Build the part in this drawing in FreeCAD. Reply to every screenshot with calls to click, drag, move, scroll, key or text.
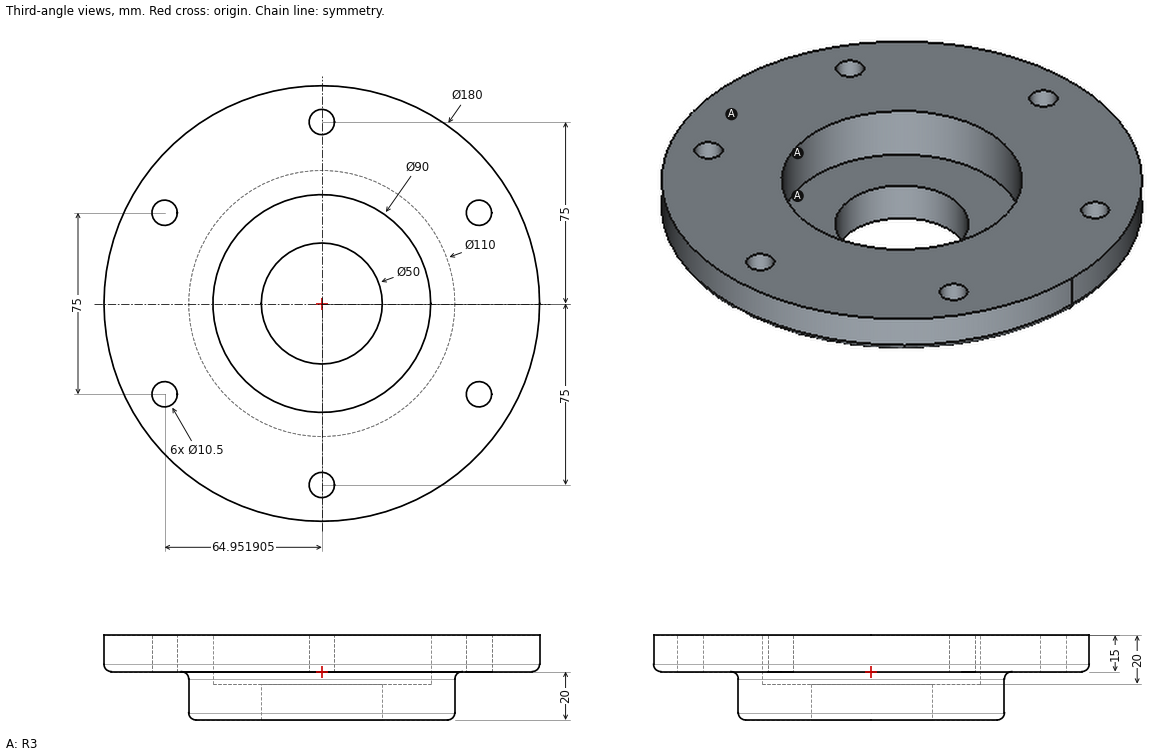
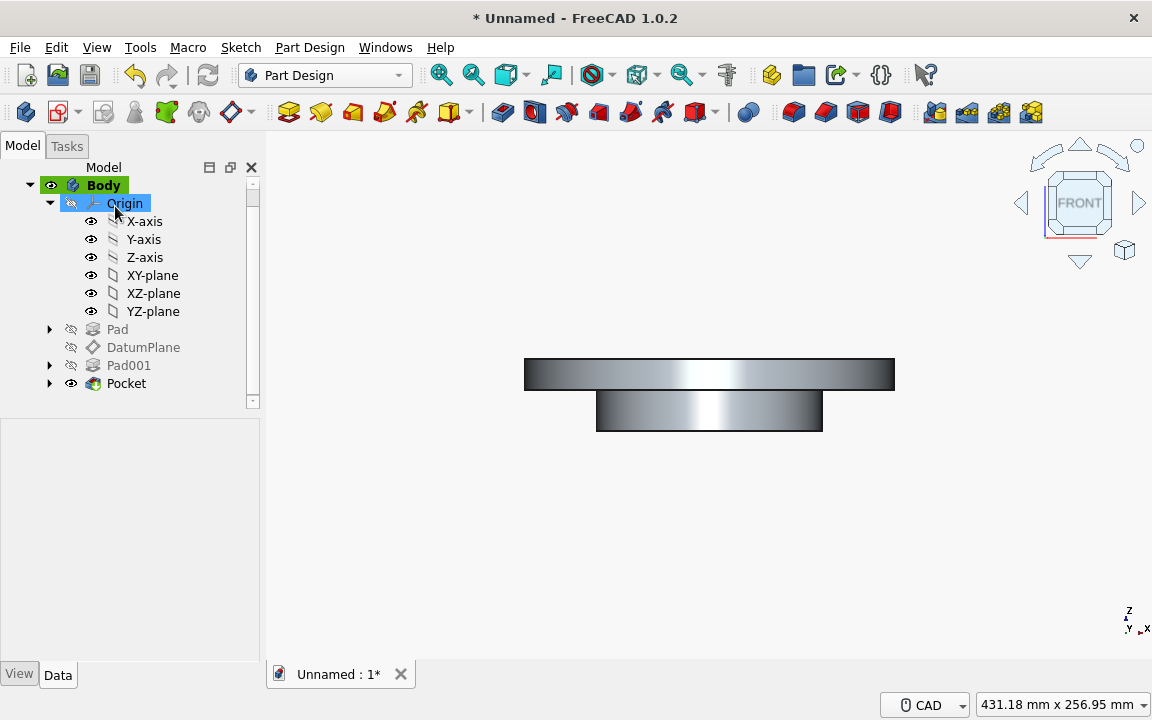
click(559, 389)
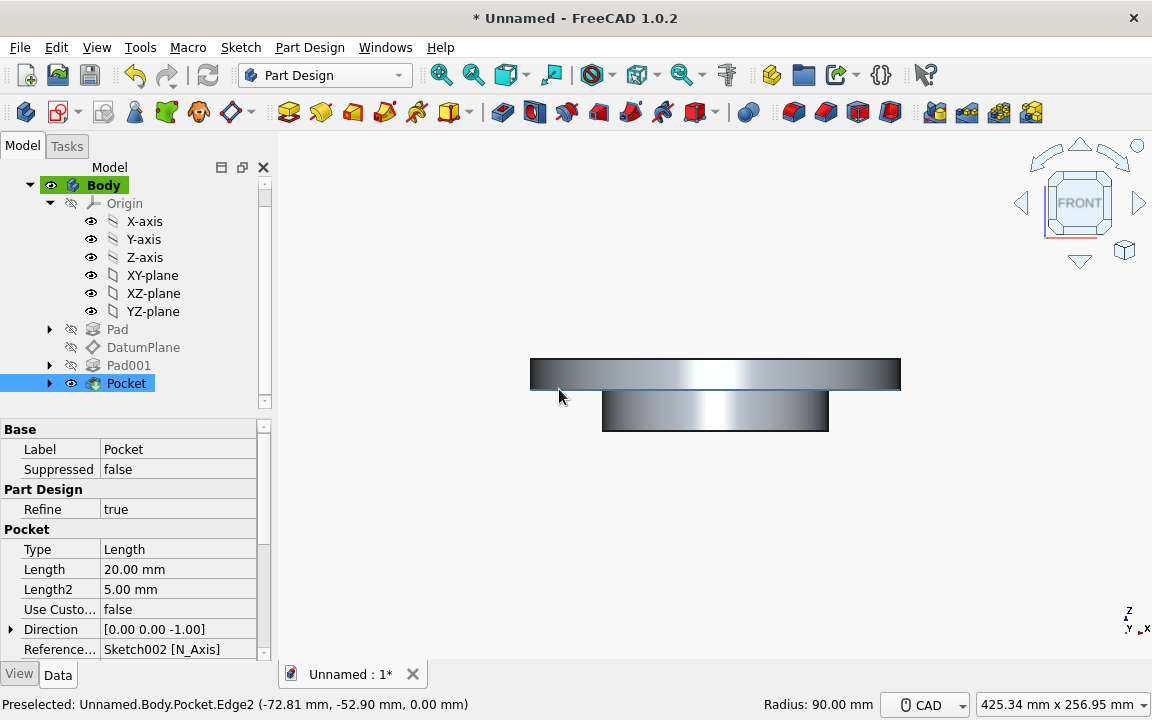
click(624, 430, ctrl)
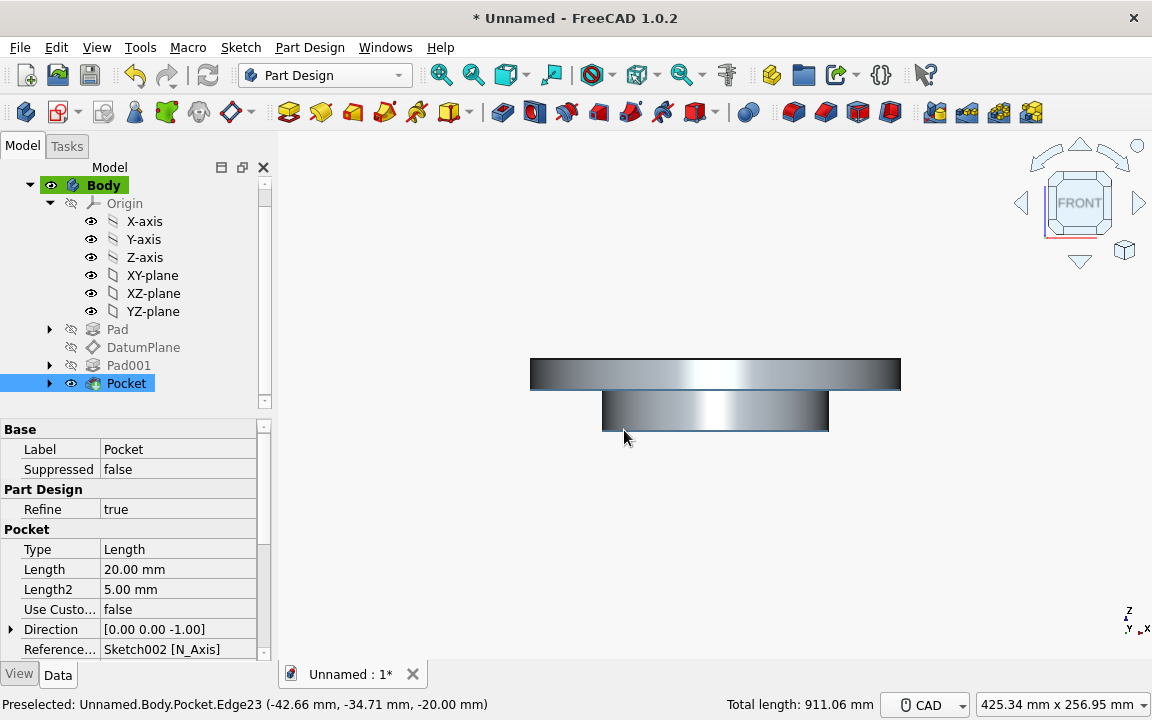
key(3)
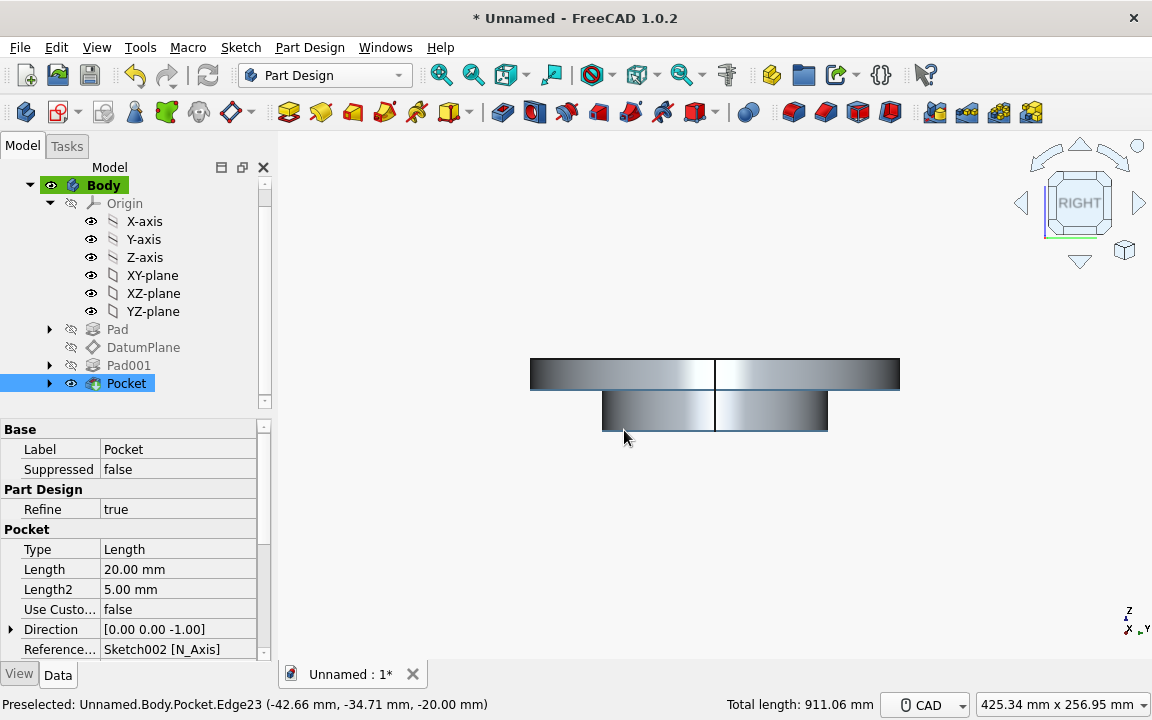
key(v)
key(f)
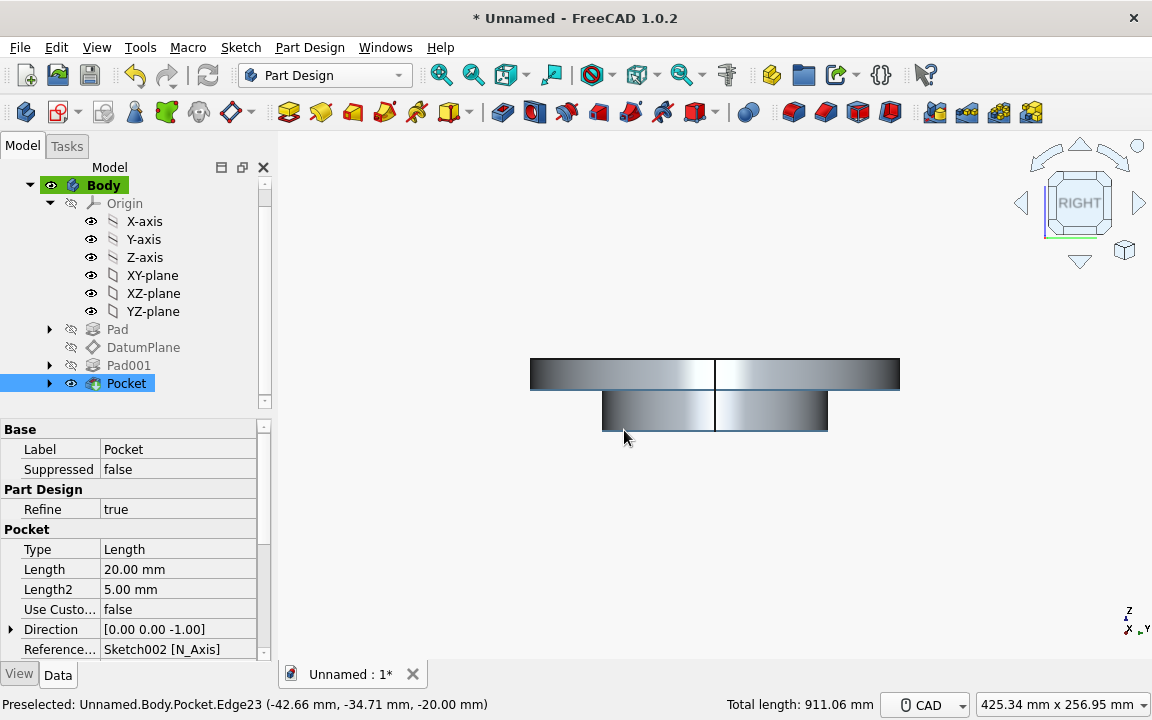
key(5)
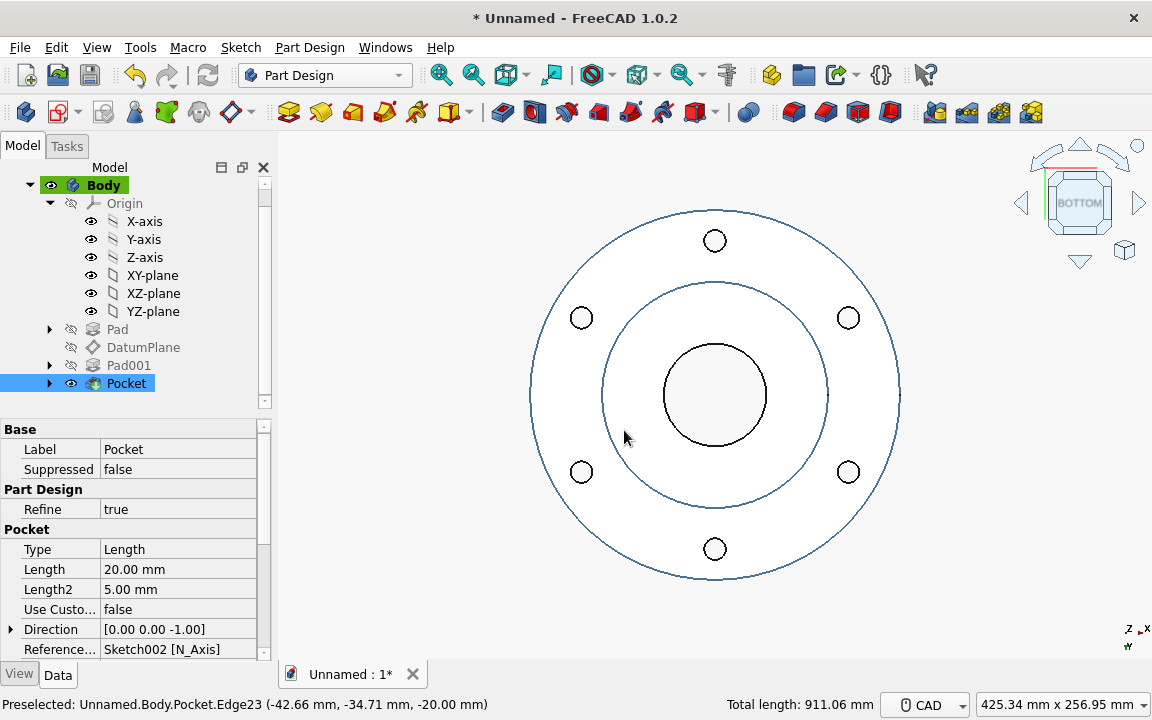
key(4)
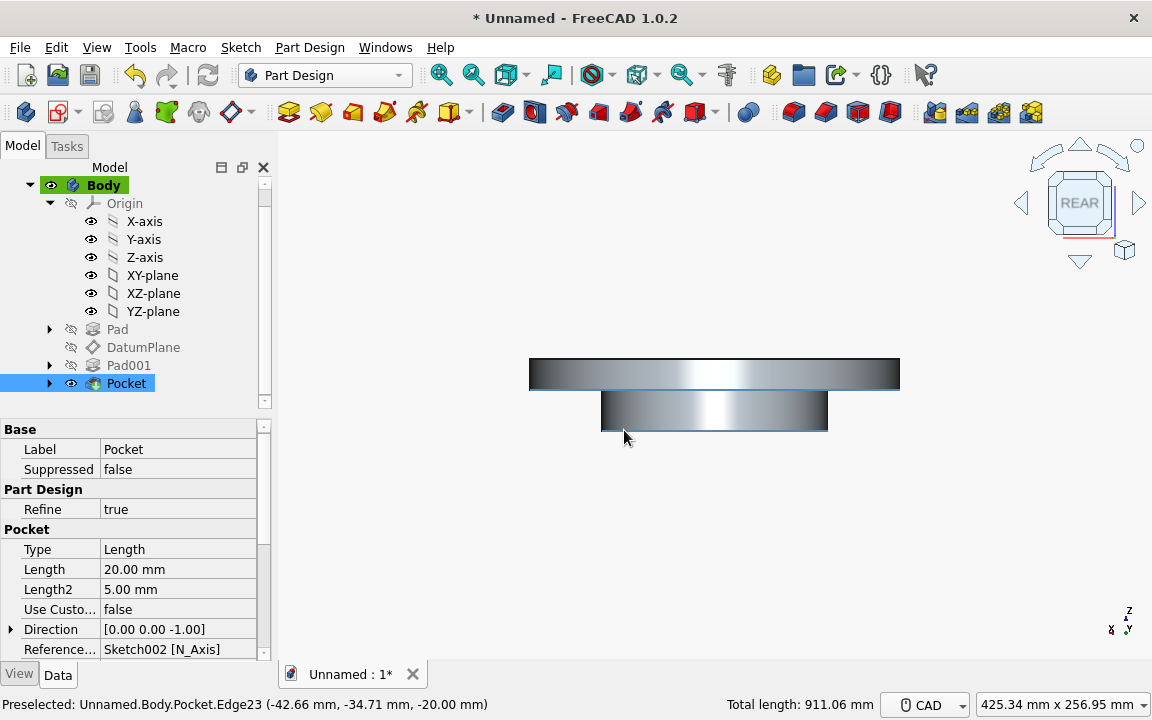
key(v)
key(f)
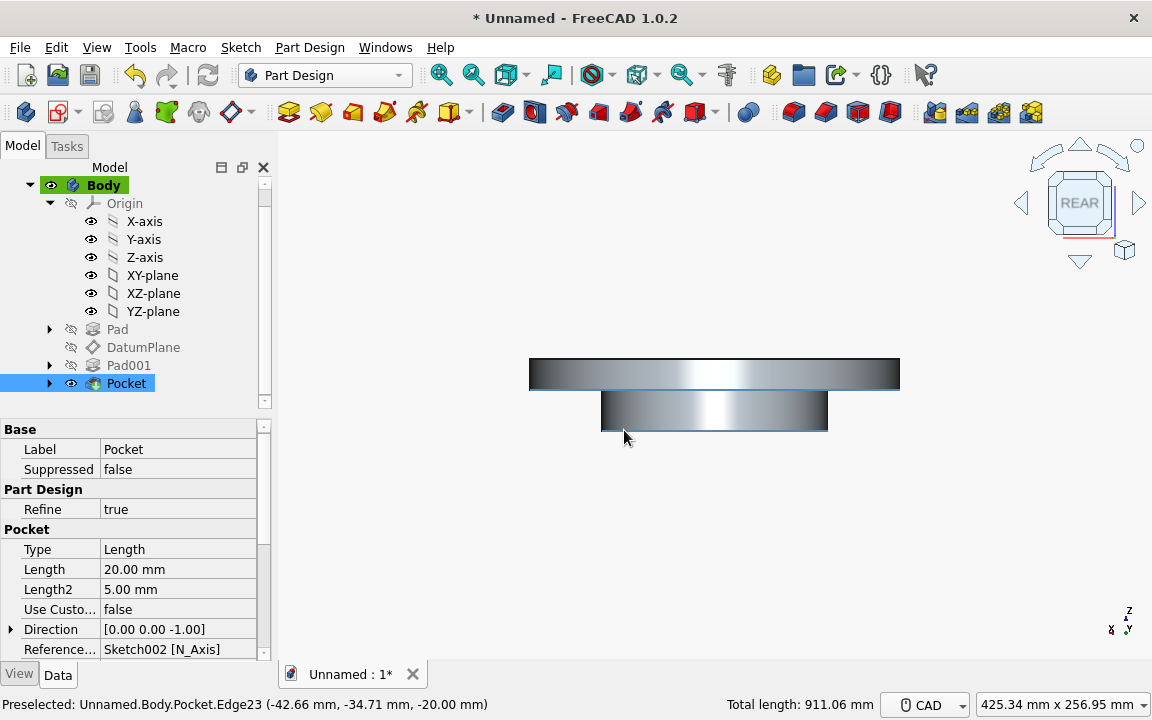
key(6)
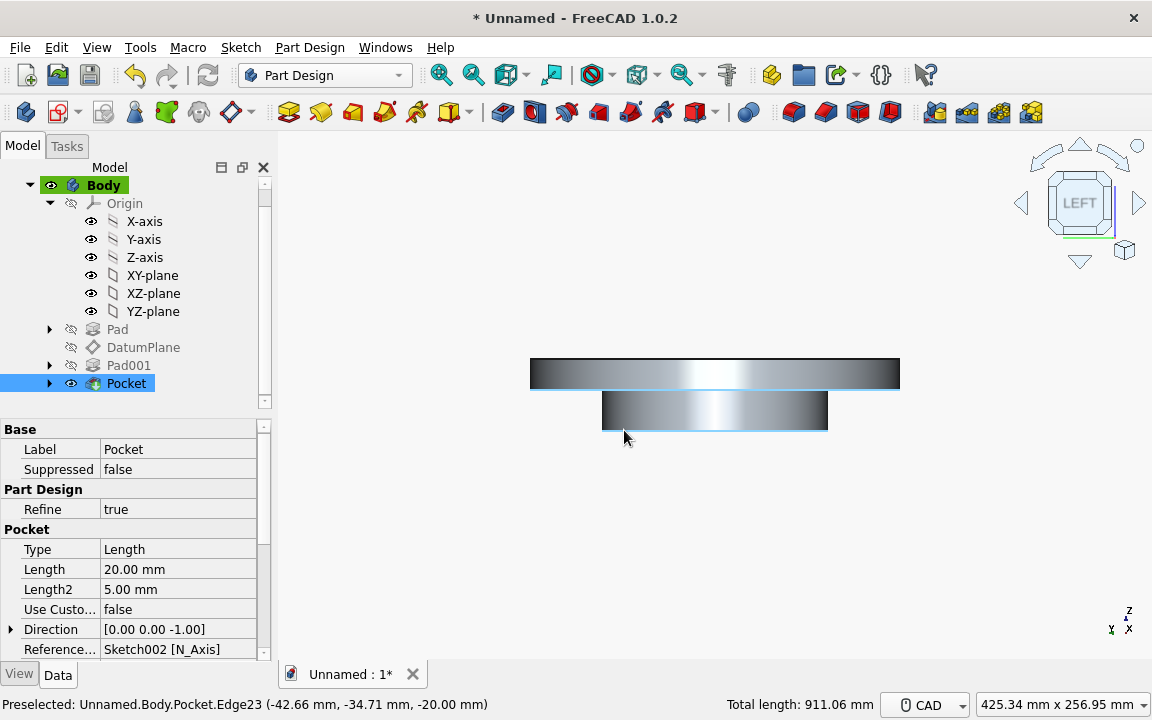
key(v)
key(f)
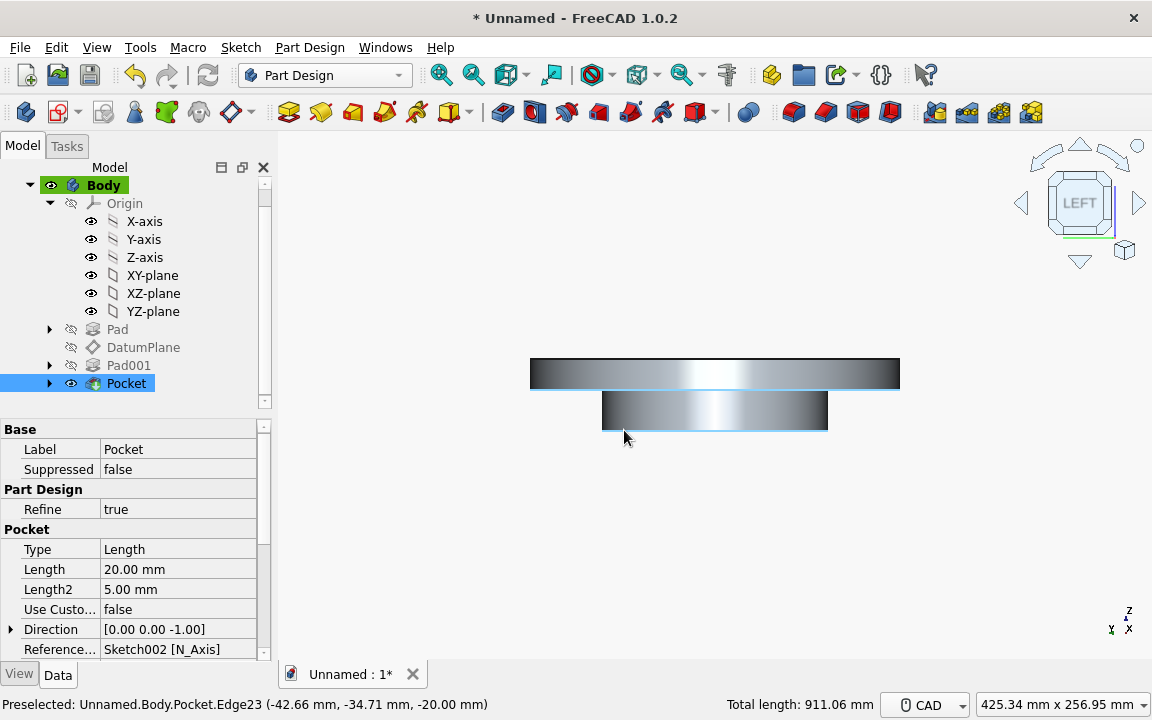
key(v)
key(3)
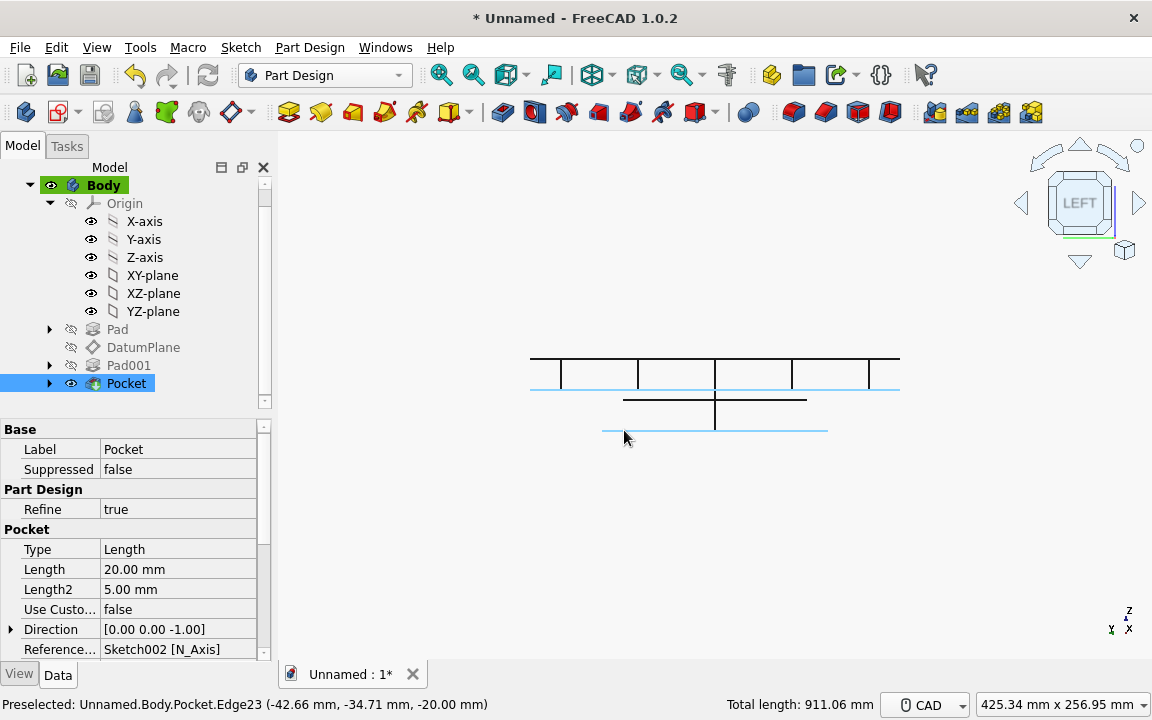
key(0)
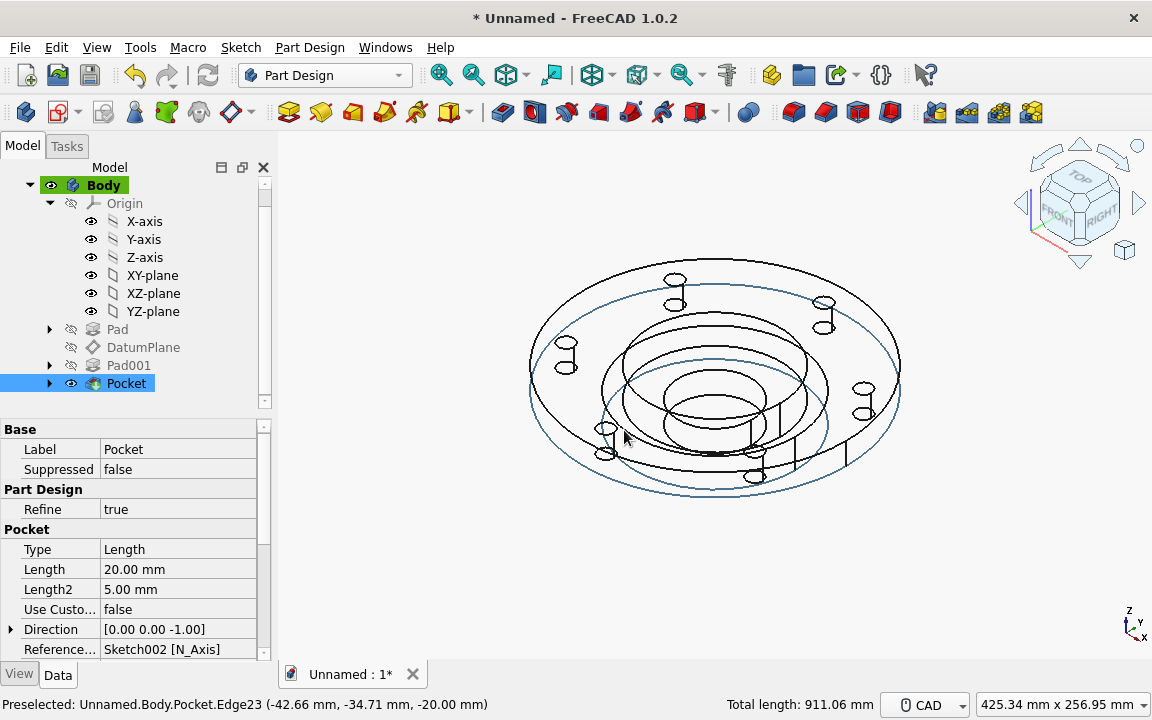
click(697, 325, ctrl)